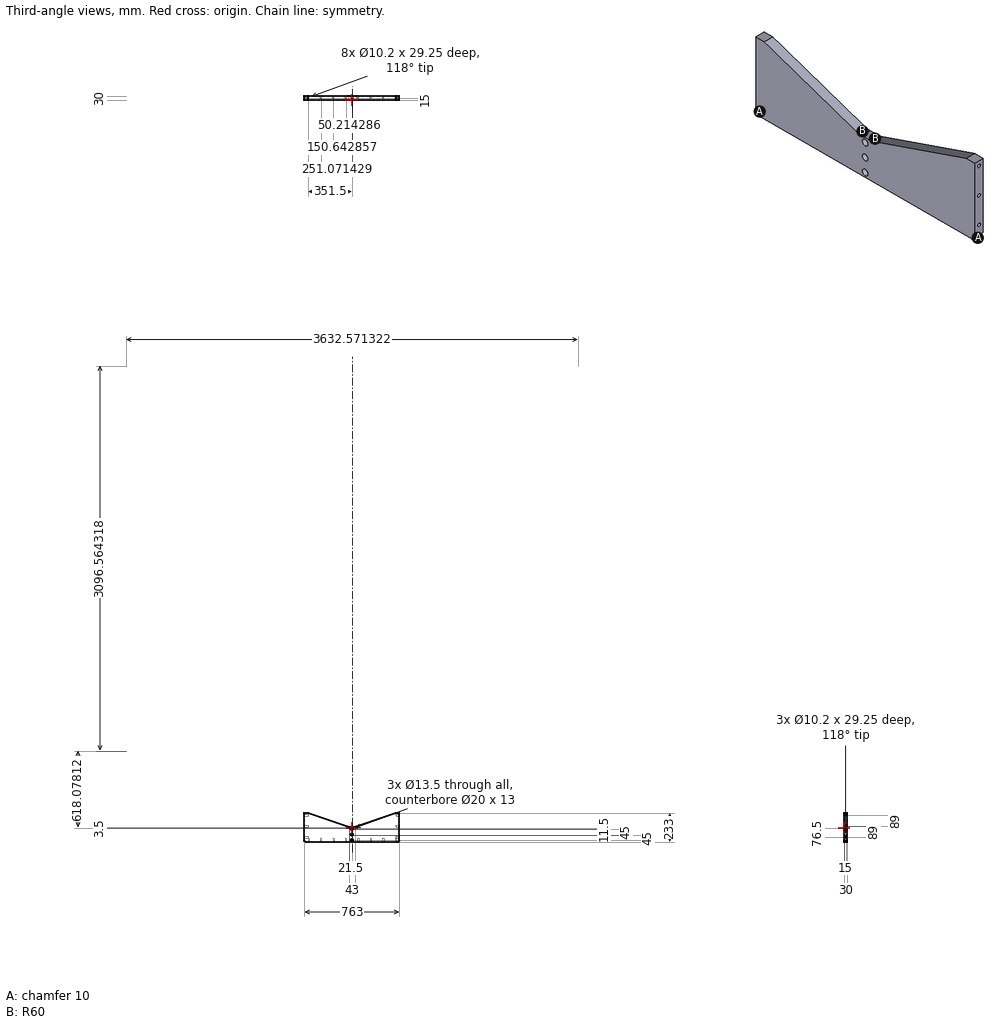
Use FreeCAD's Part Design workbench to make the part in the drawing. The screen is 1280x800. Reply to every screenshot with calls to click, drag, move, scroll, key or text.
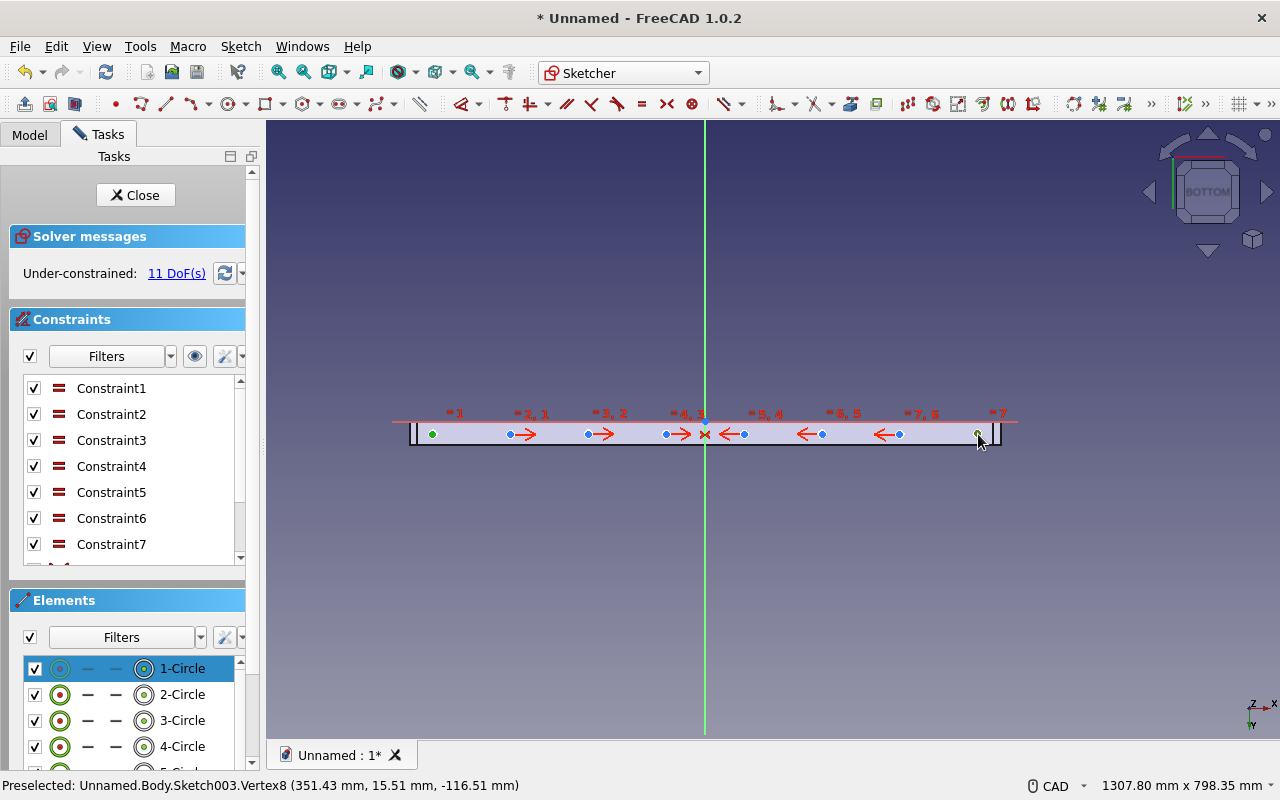
click(705, 671)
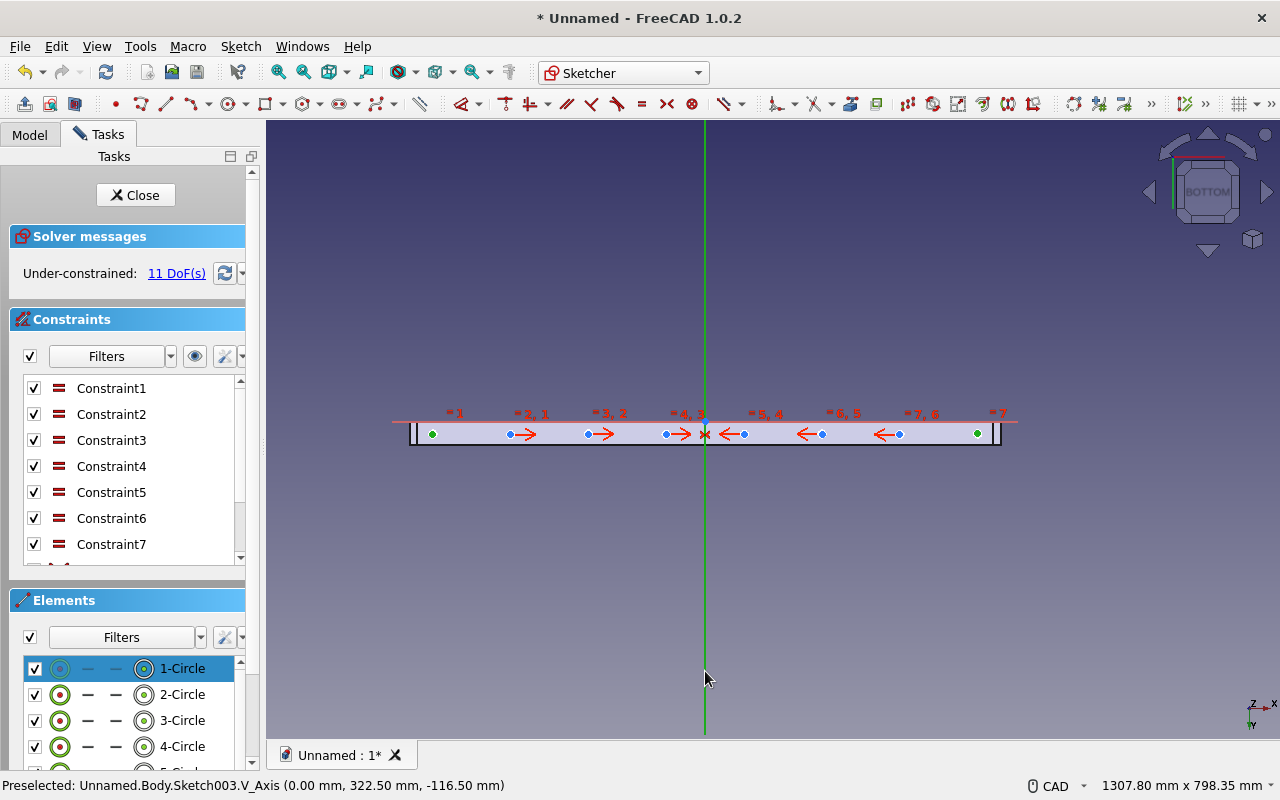
key(s)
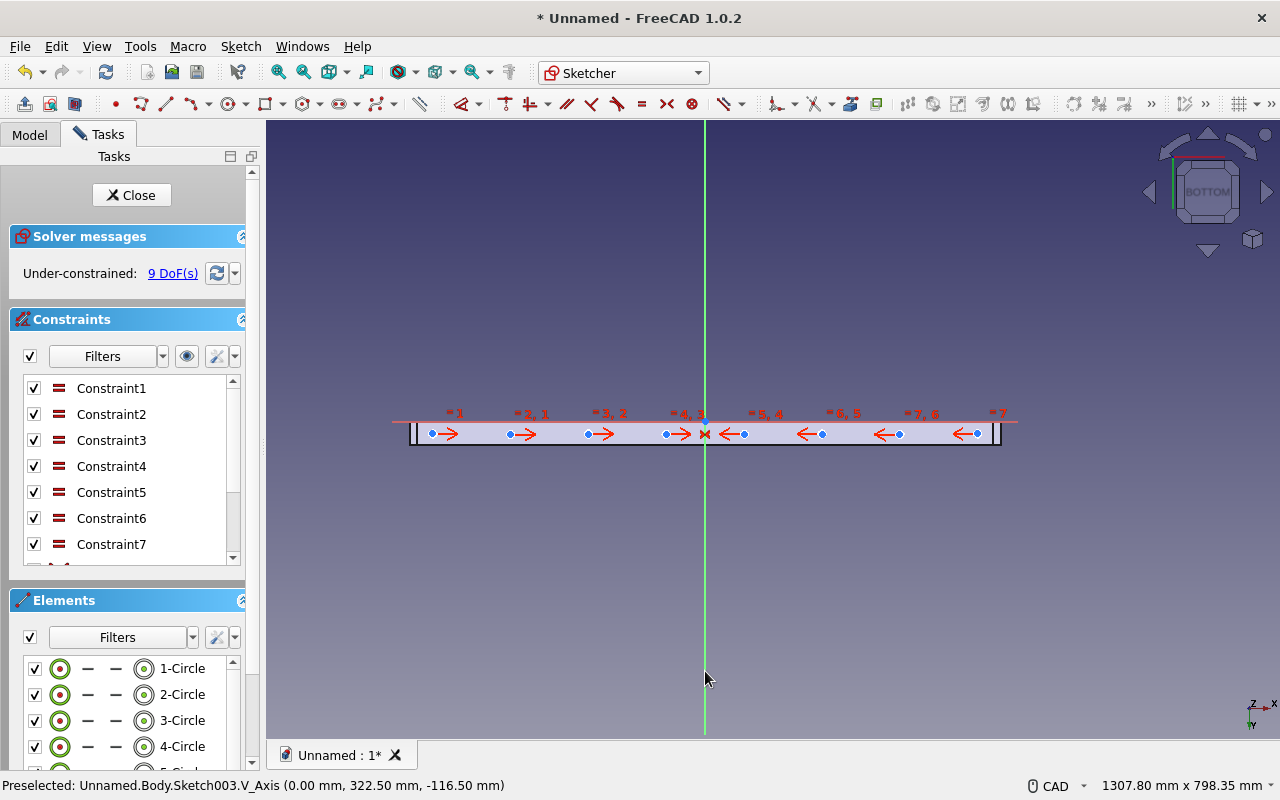
key(d)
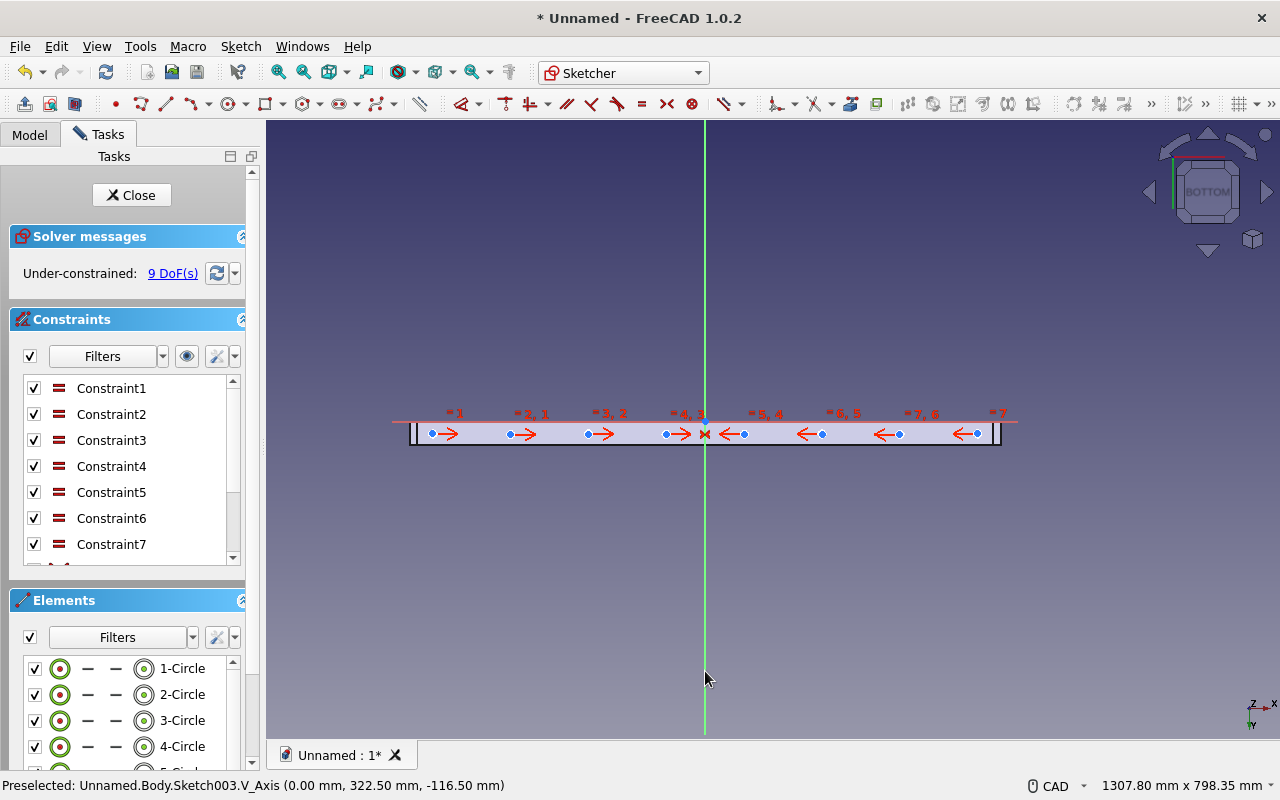
scroll(429, 434, up, 9)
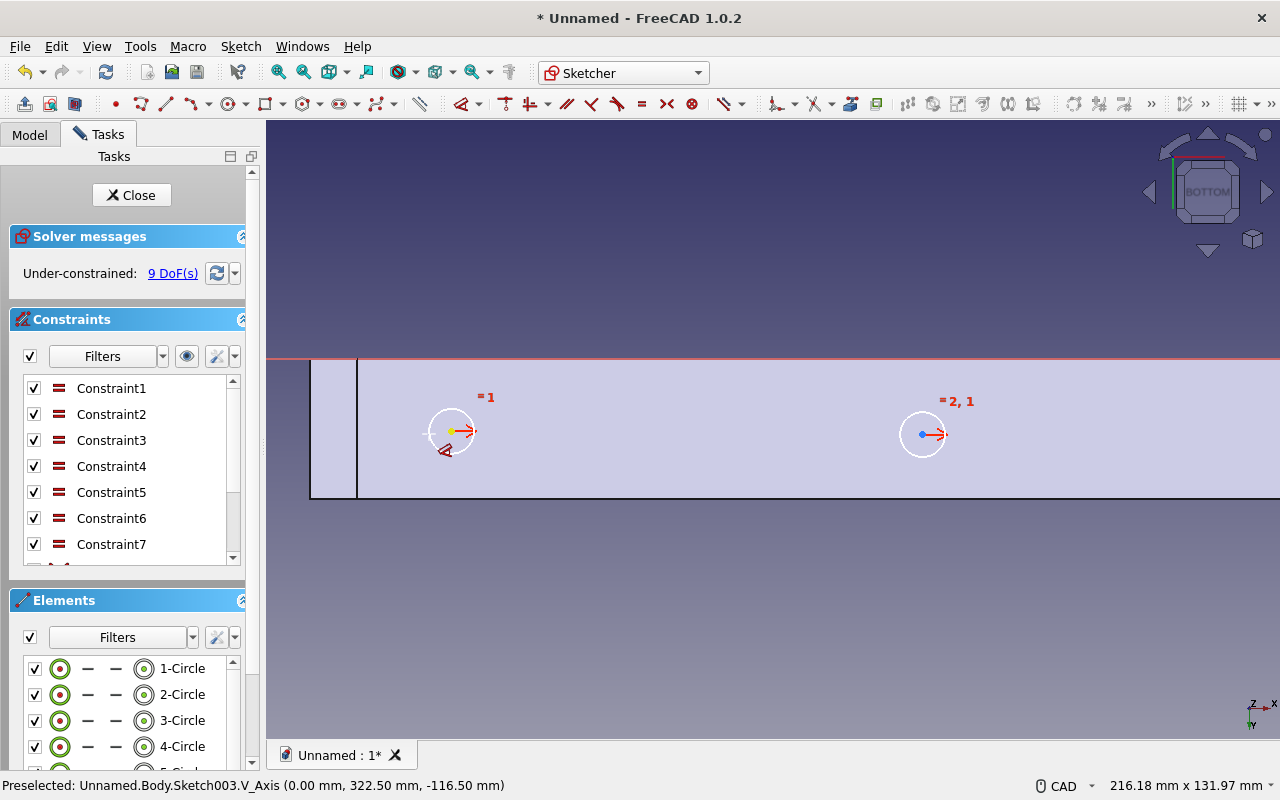
click(429, 431)
click(397, 431)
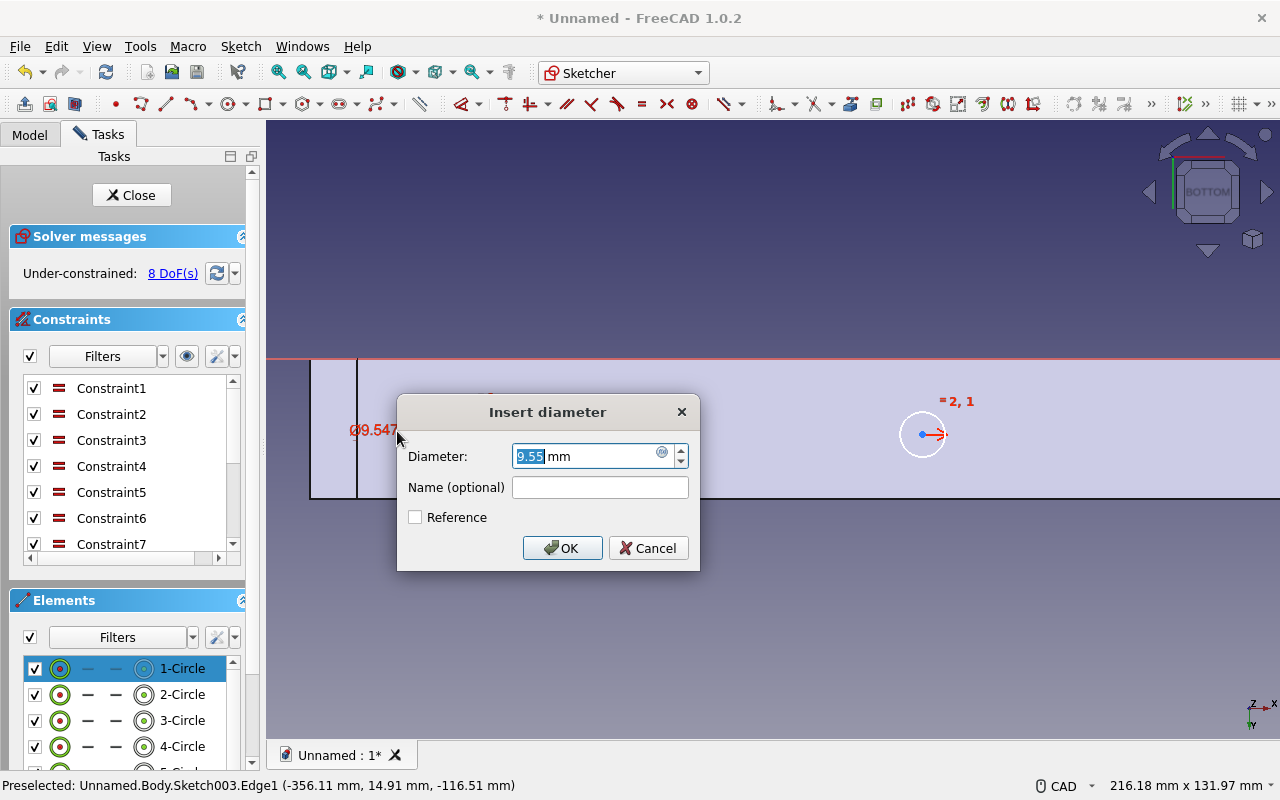
text(10.2)
key(Return)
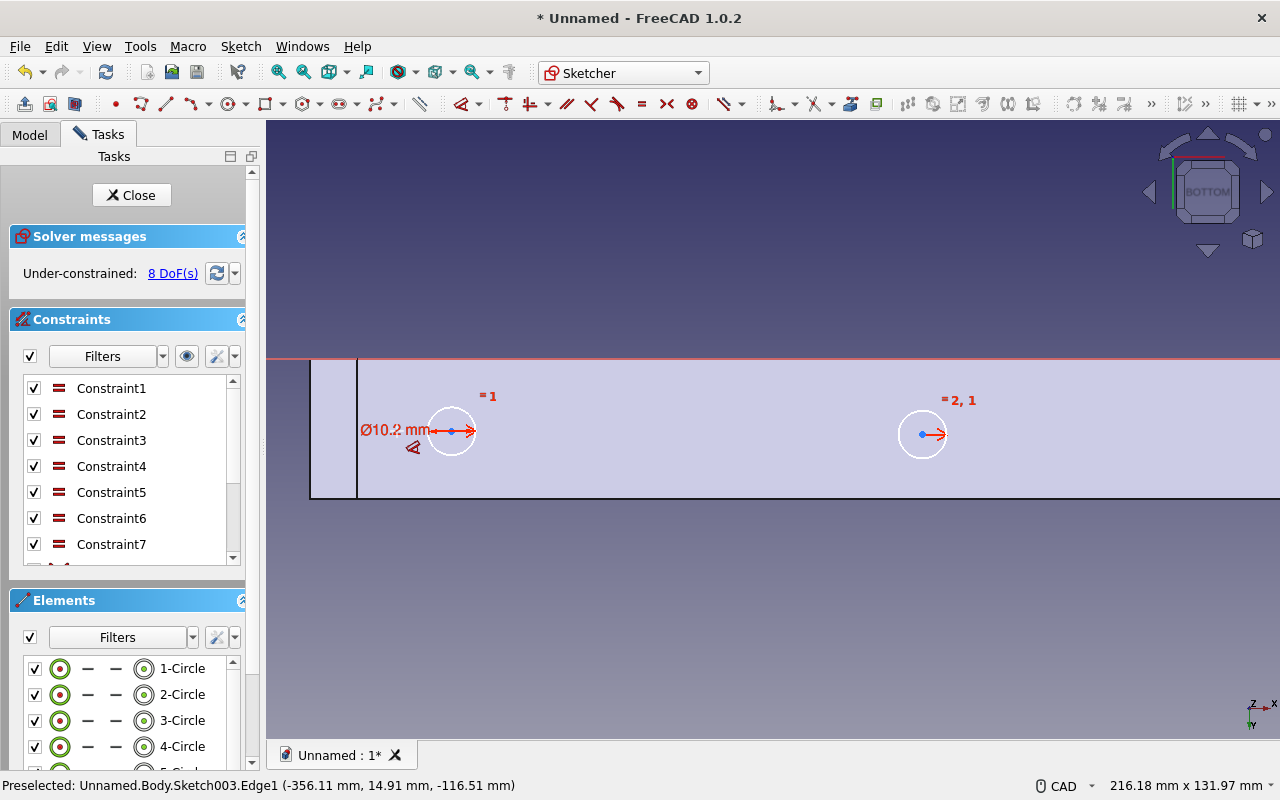
click(452, 431)
click(418, 395)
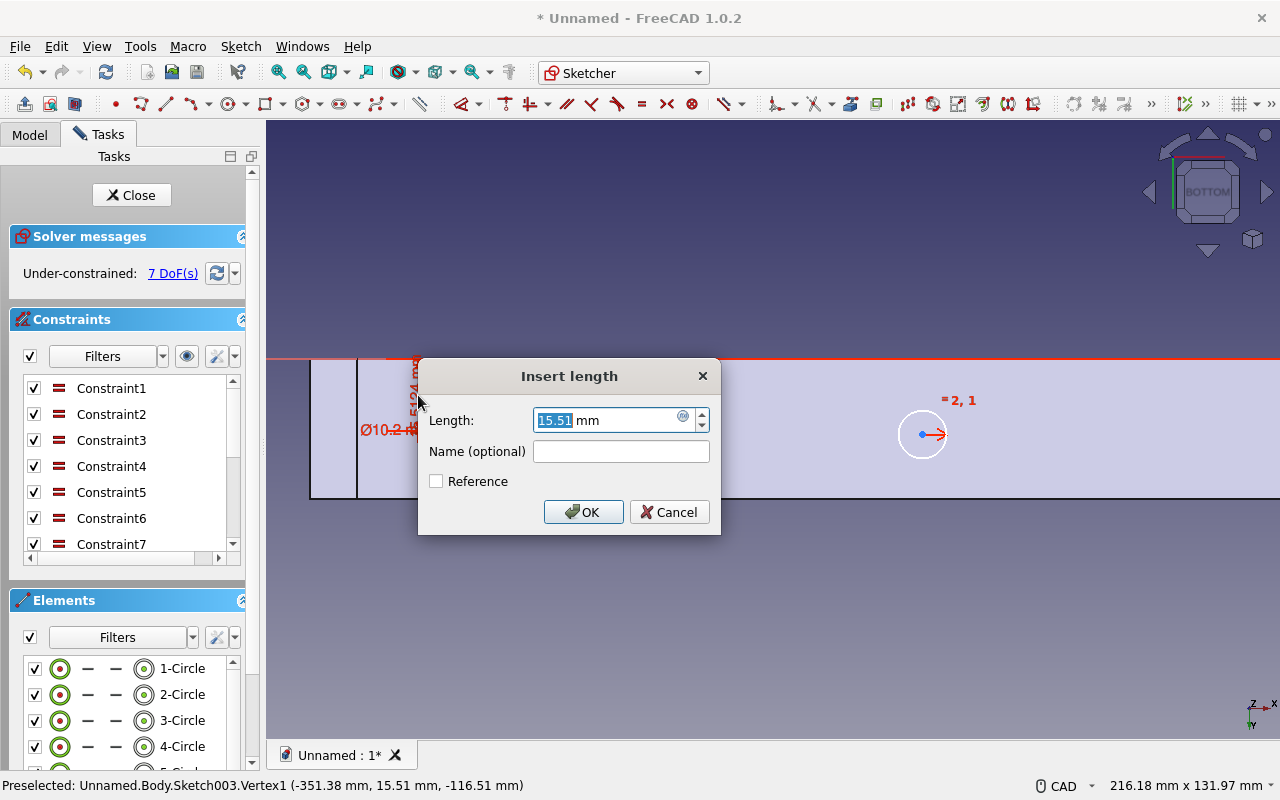
text(15)
key(Return)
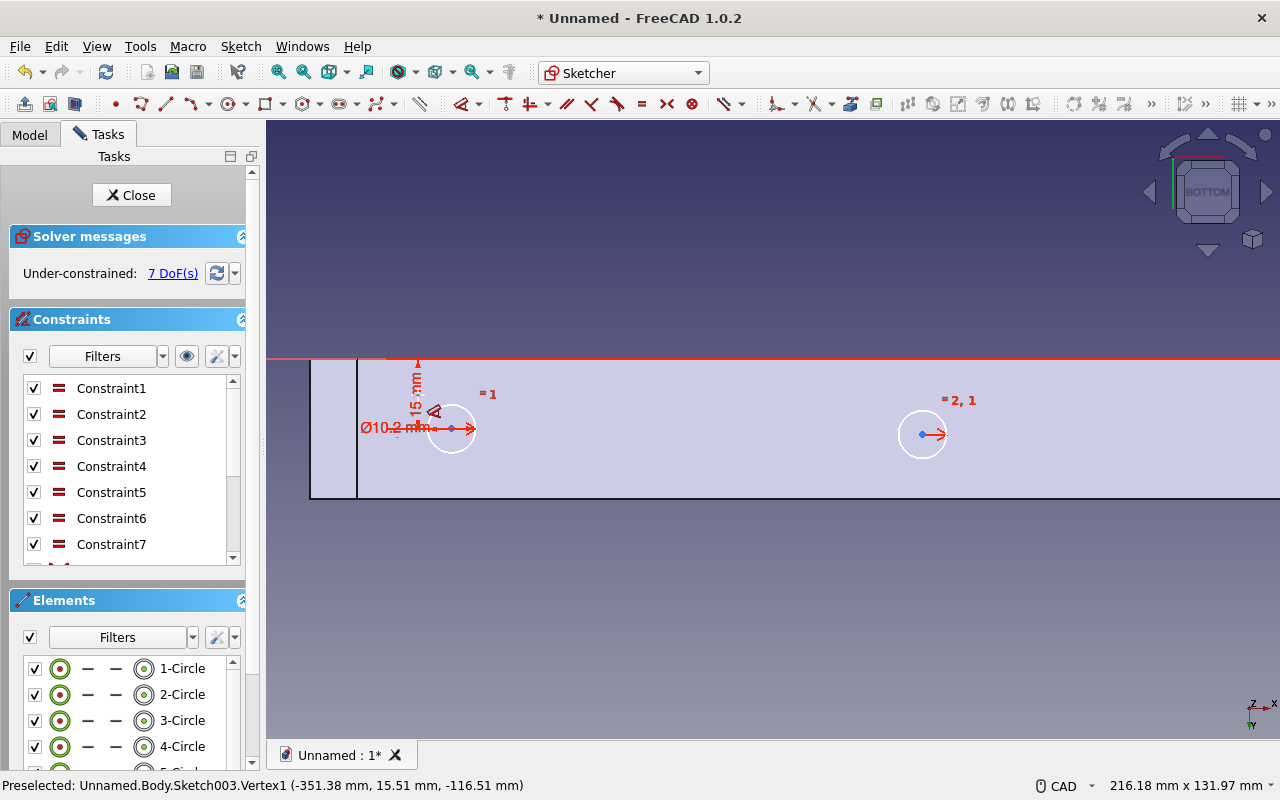
click(923, 435)
click(889, 397)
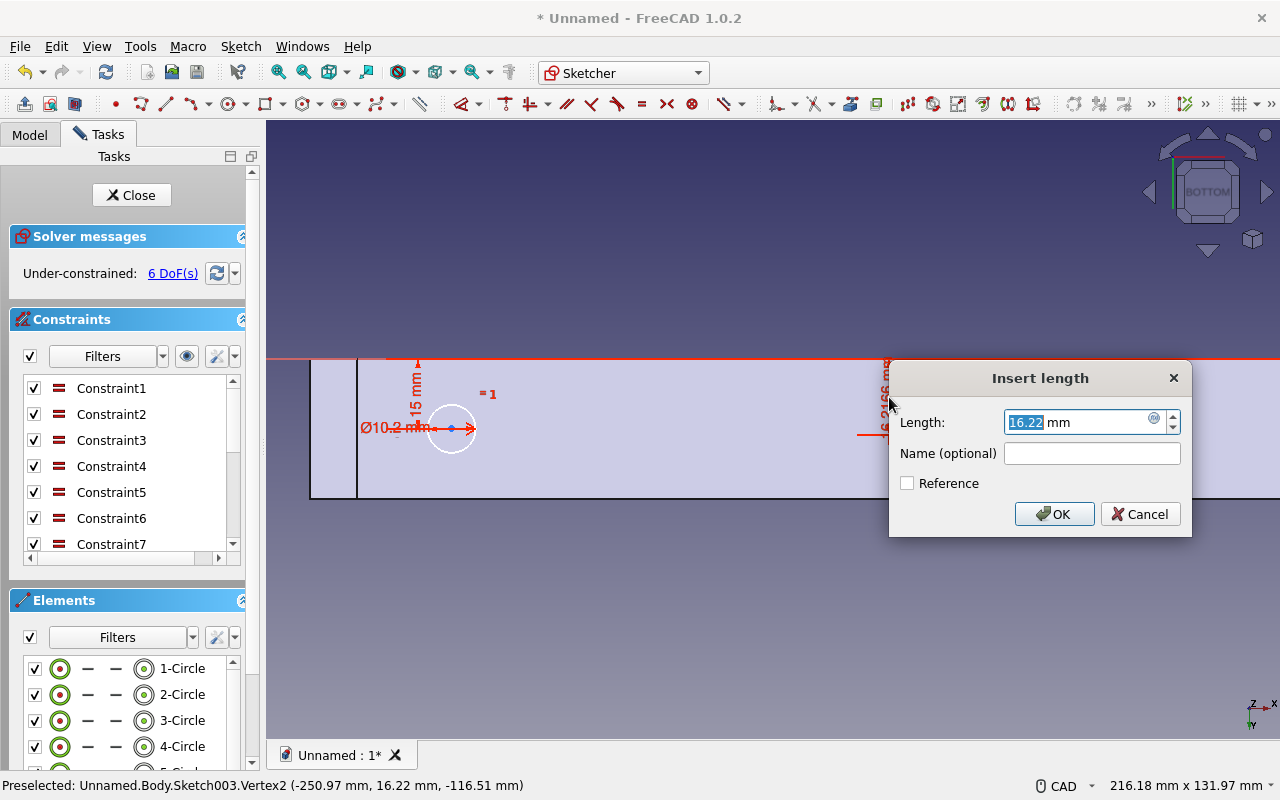
text(15)
key(Return)